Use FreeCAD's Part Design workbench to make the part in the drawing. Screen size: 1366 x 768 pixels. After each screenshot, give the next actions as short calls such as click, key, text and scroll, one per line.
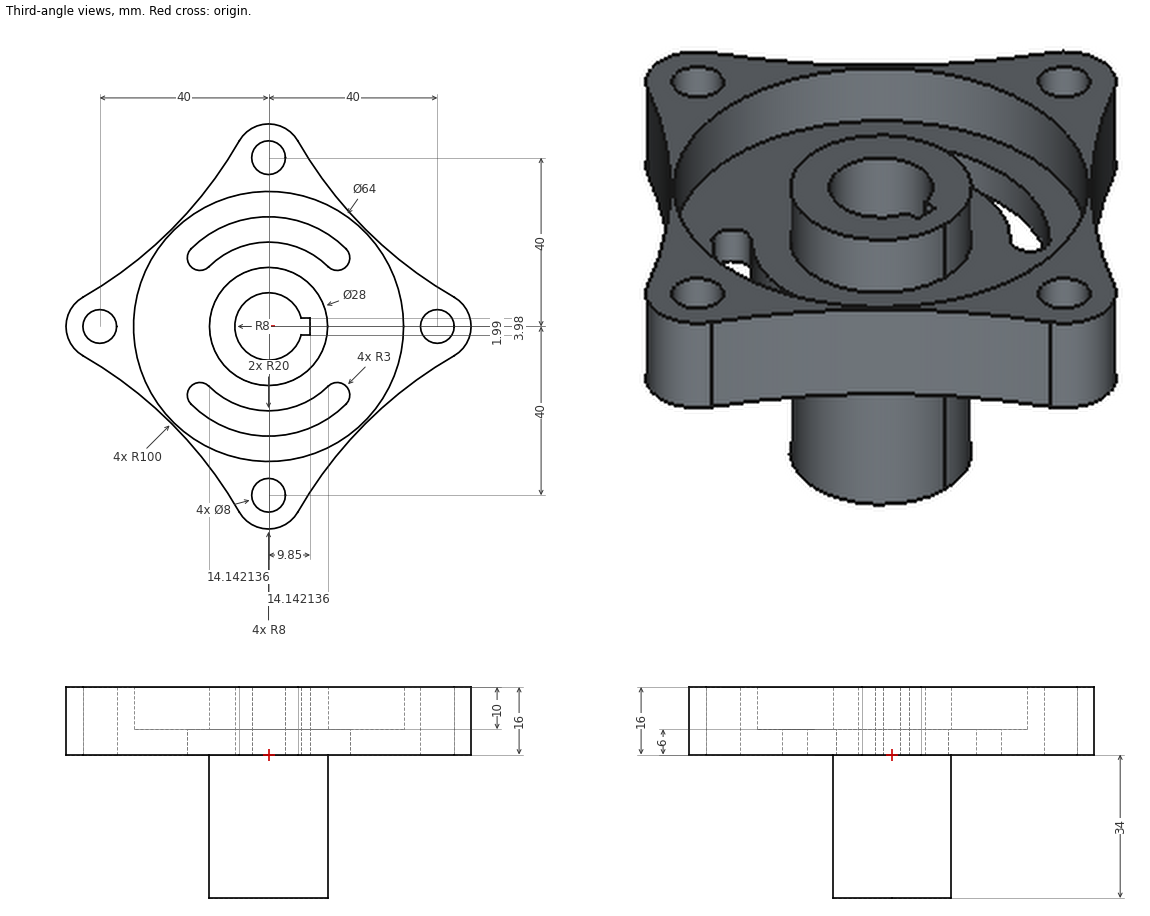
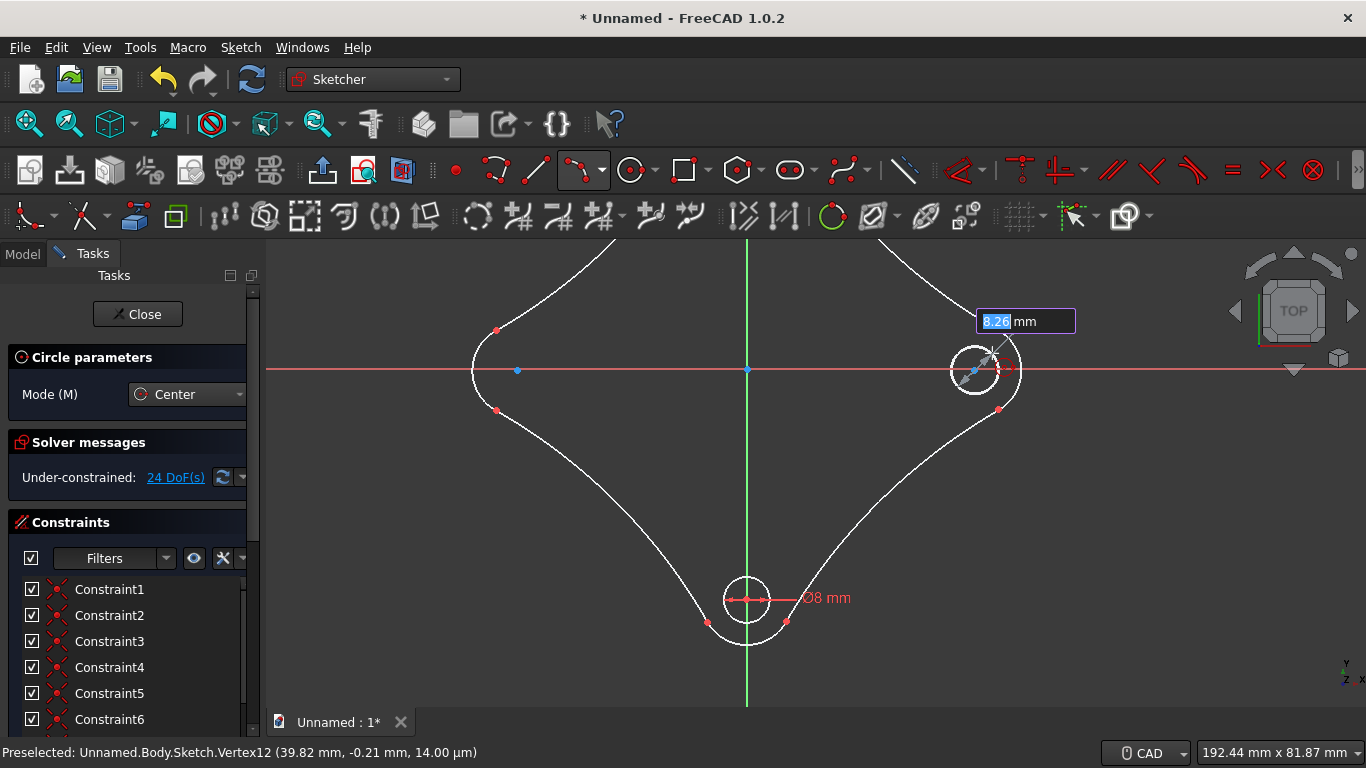
text(8)
key(Return)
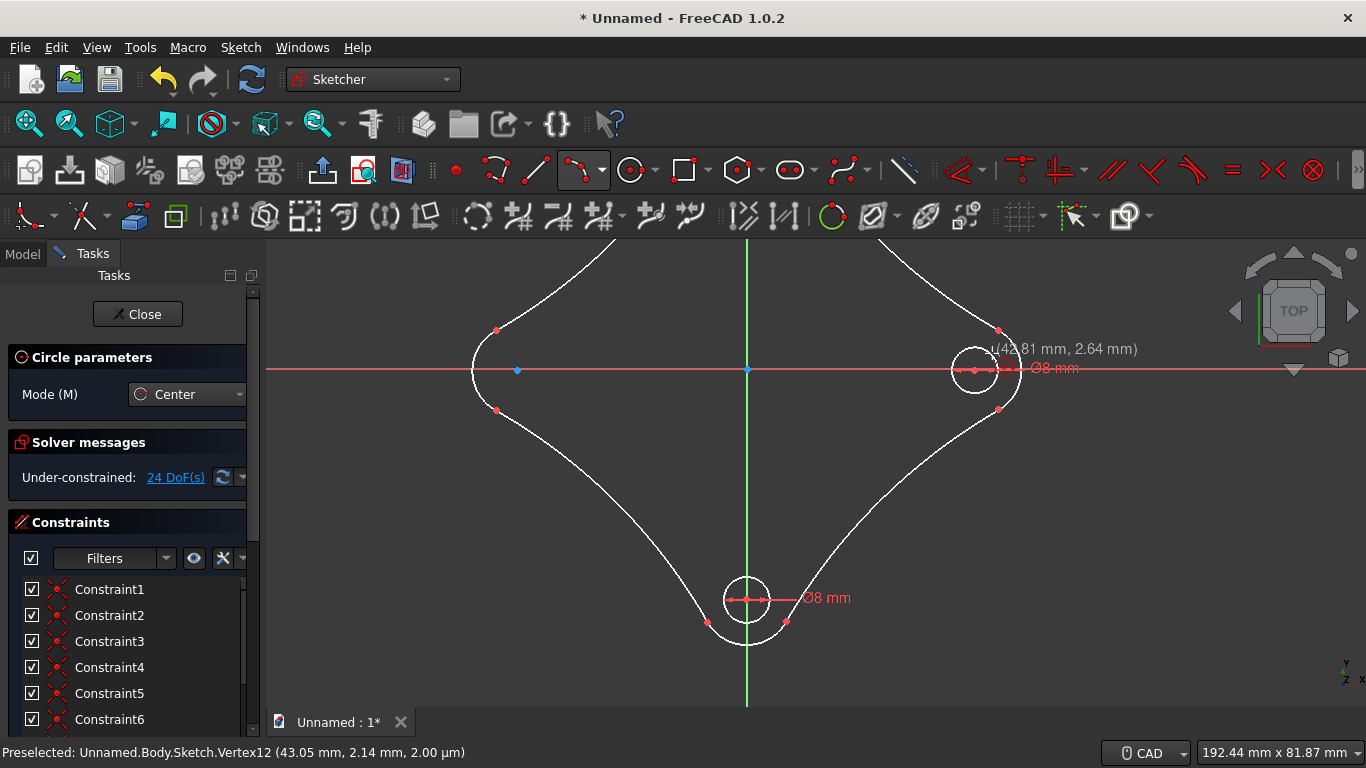
click(519, 369)
move(535, 353)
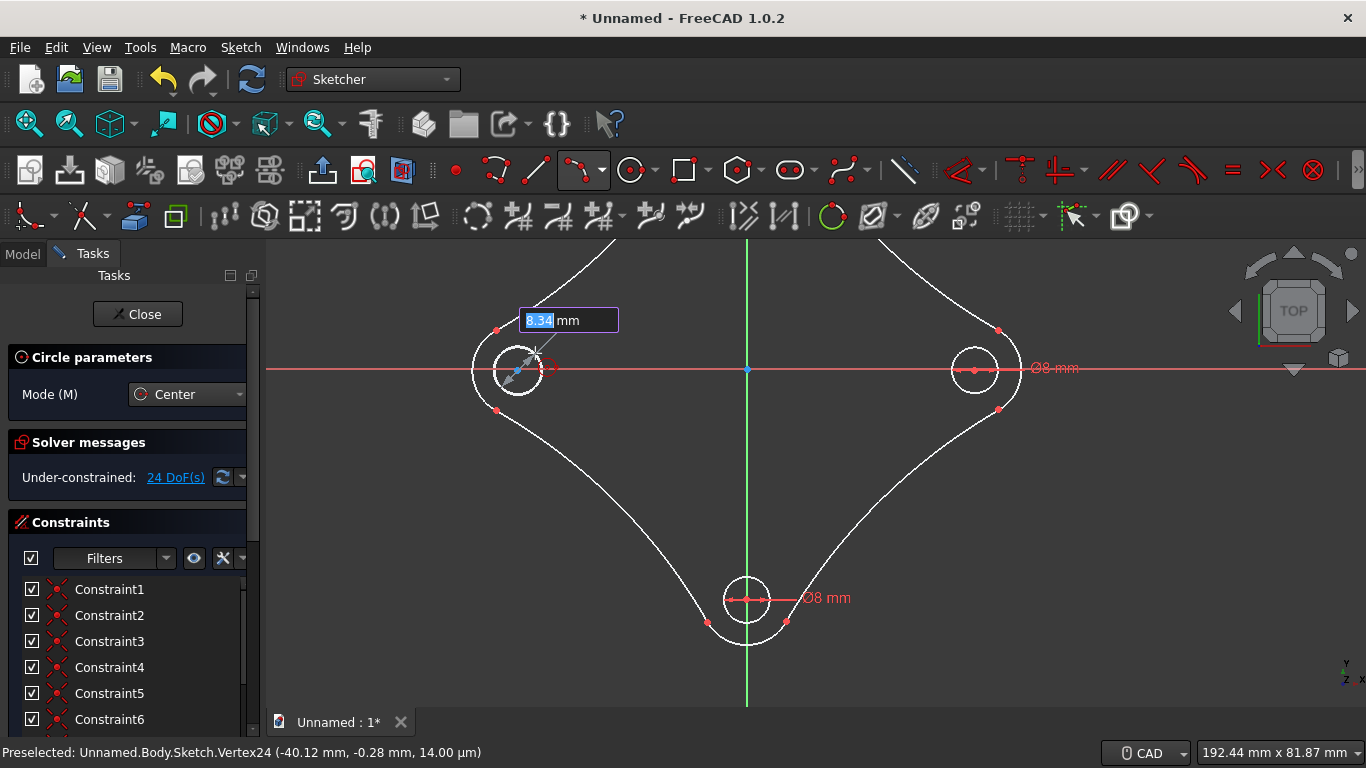
text(8)
key(Return)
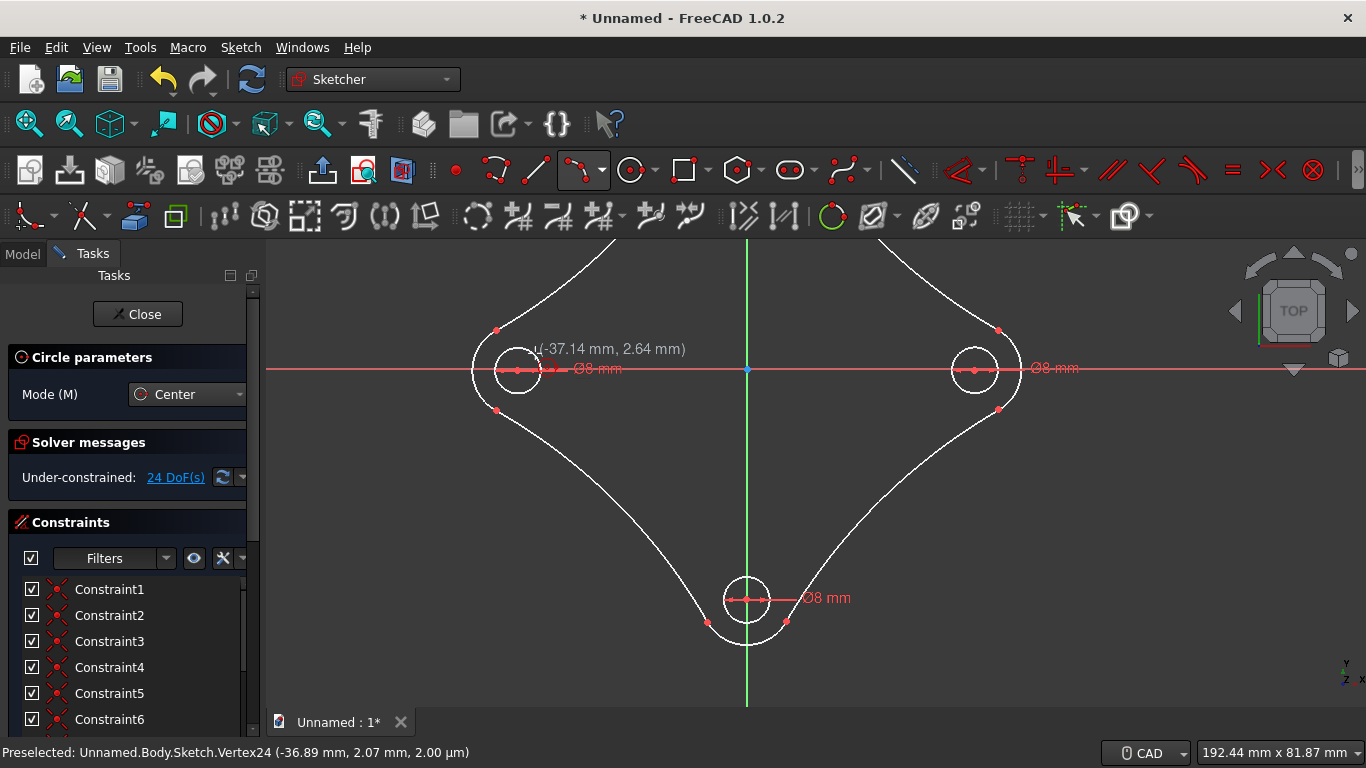
scroll(748, 599, down, 3)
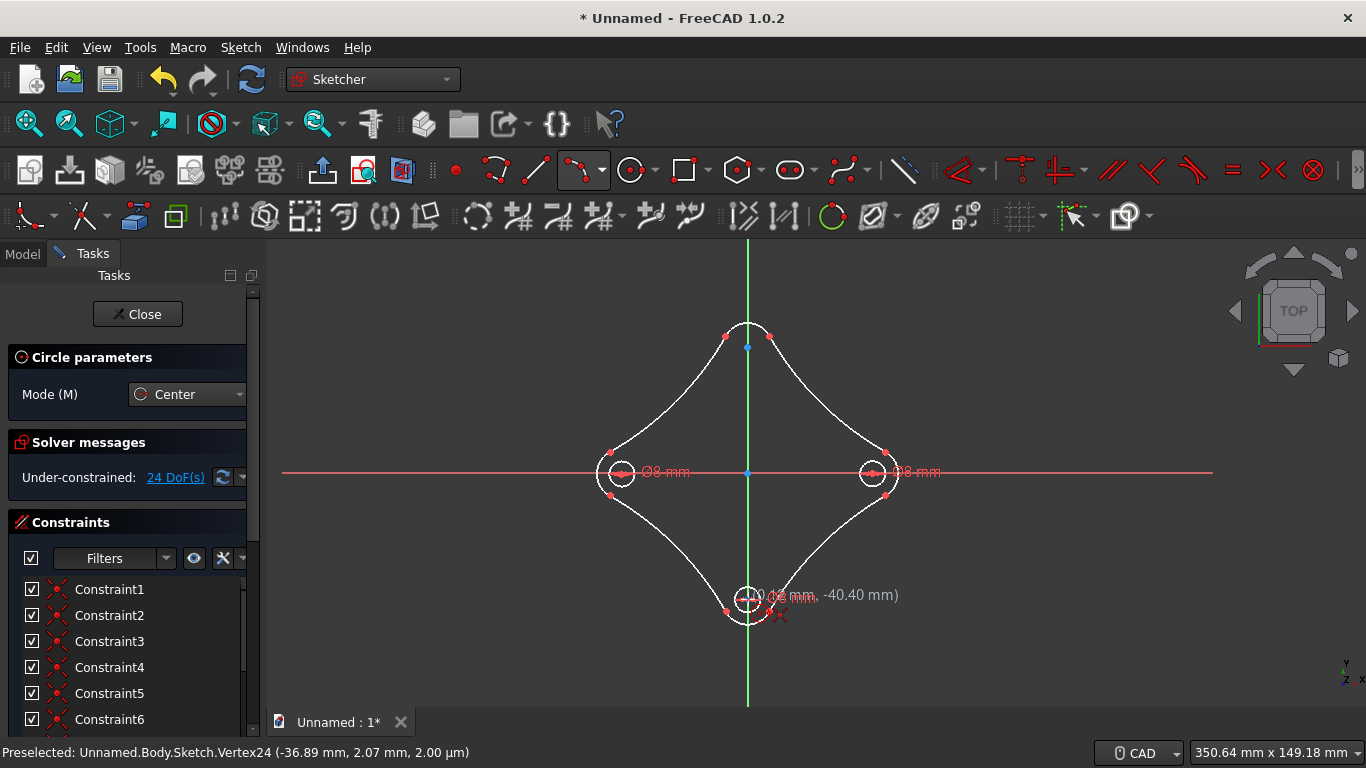
scroll(748, 348, up, 3)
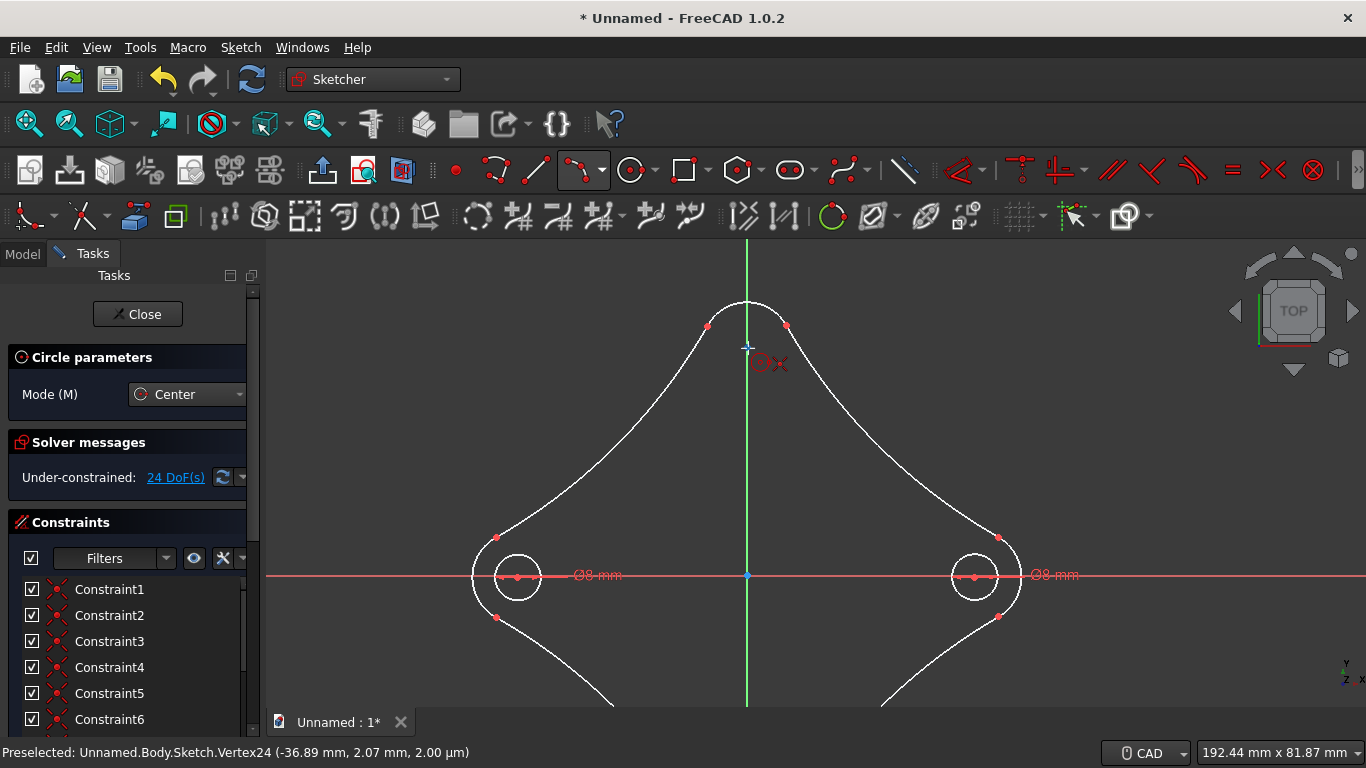
click(747, 347)
move(763, 331)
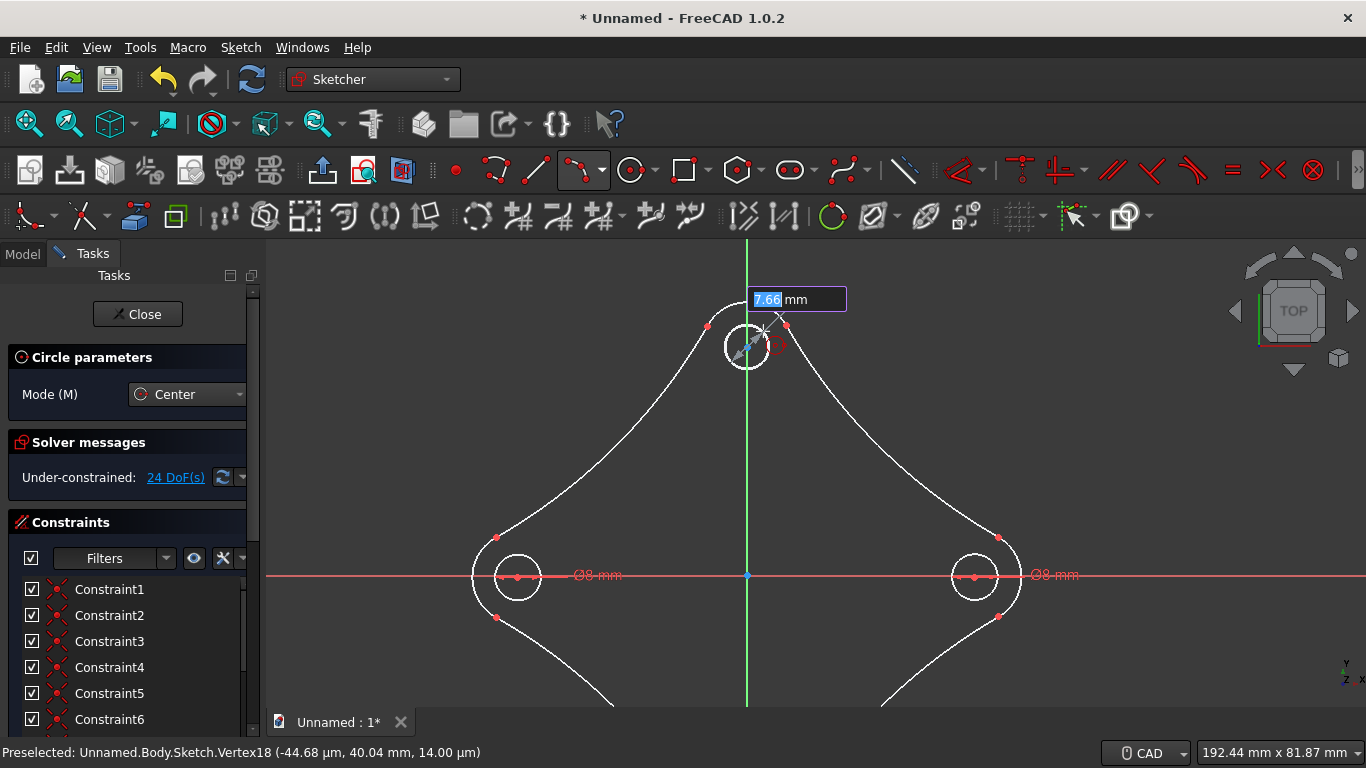
text(8)
key(Return)
key(Escape)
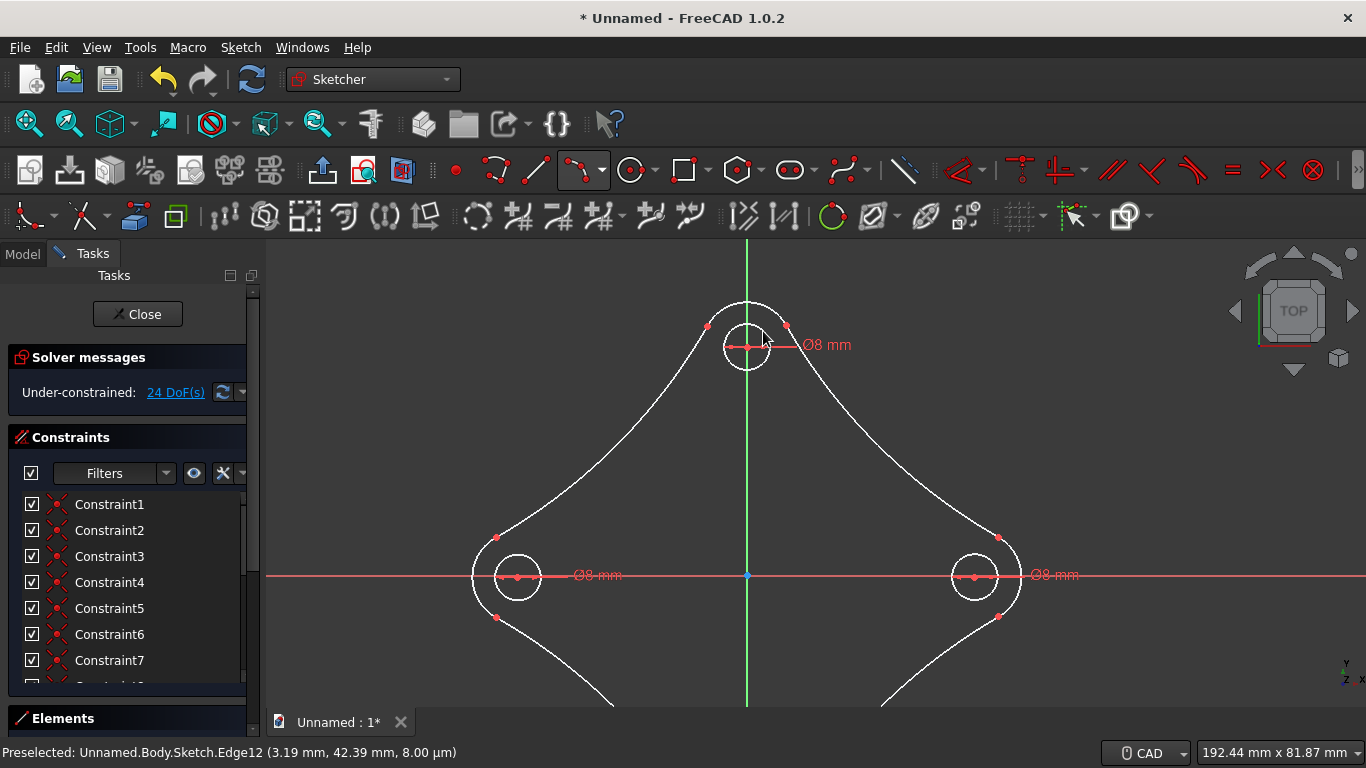
click(571, 669)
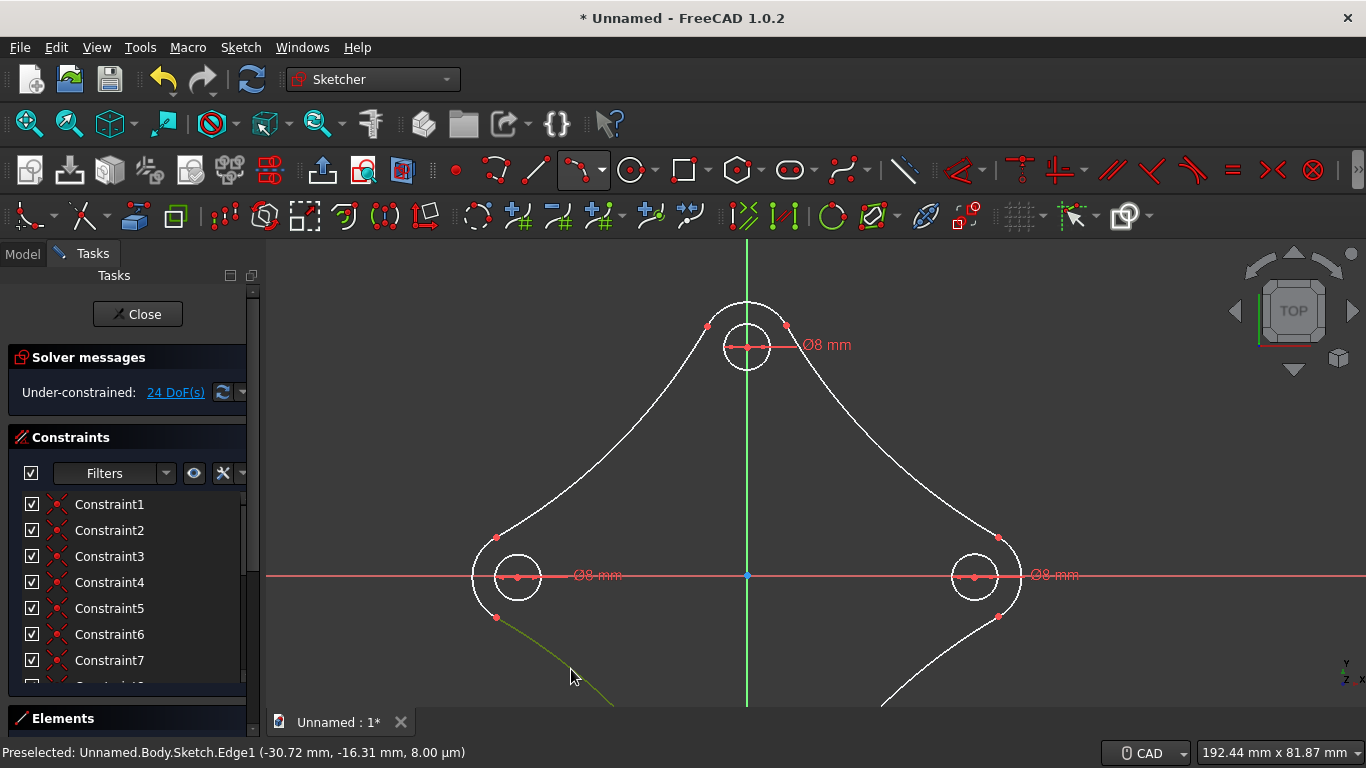
scroll(748, 348, down, 3)